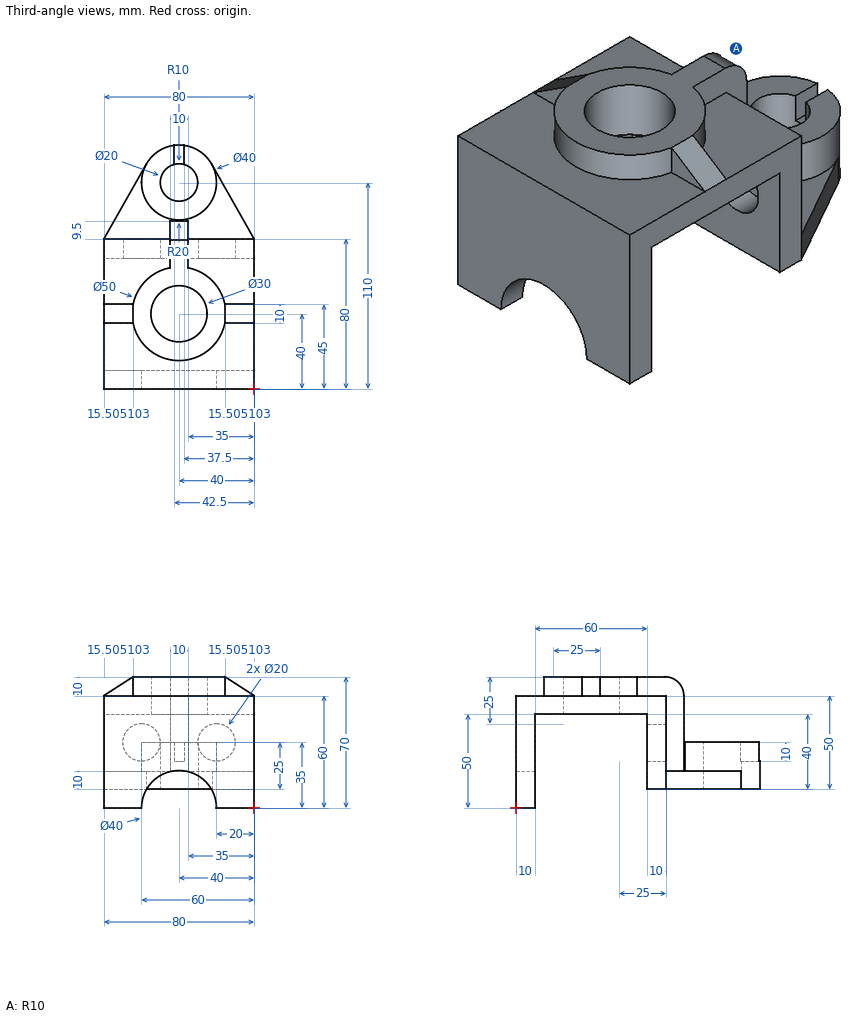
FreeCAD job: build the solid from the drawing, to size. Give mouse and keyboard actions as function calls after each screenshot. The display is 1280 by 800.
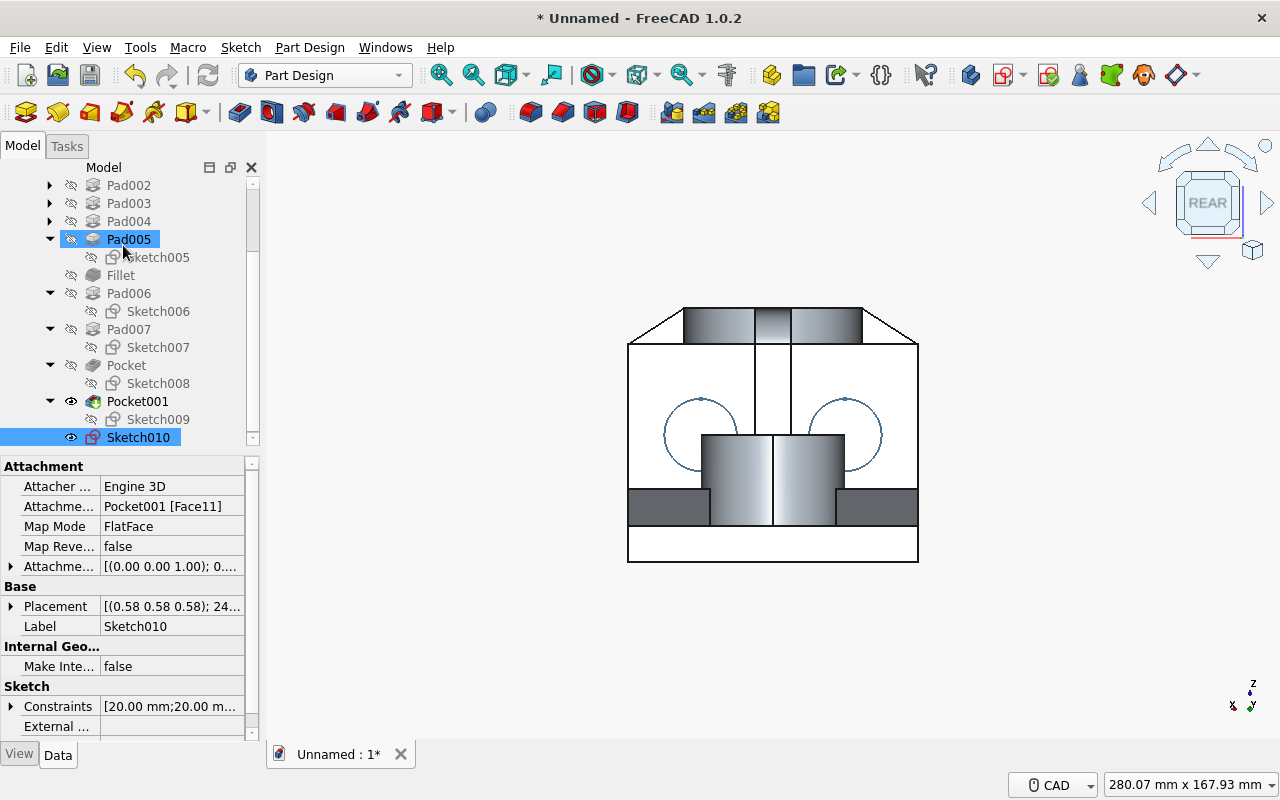
click(240, 112)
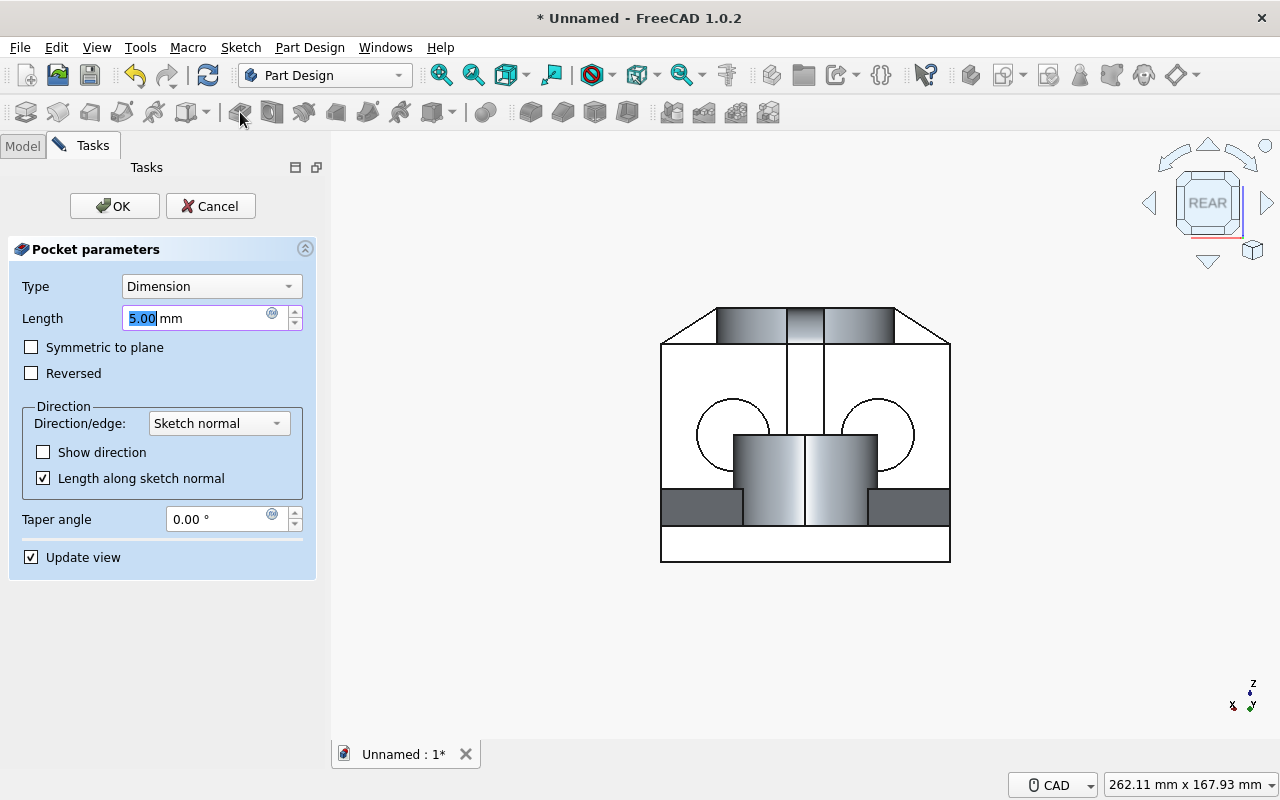
text(25)
key(Tab)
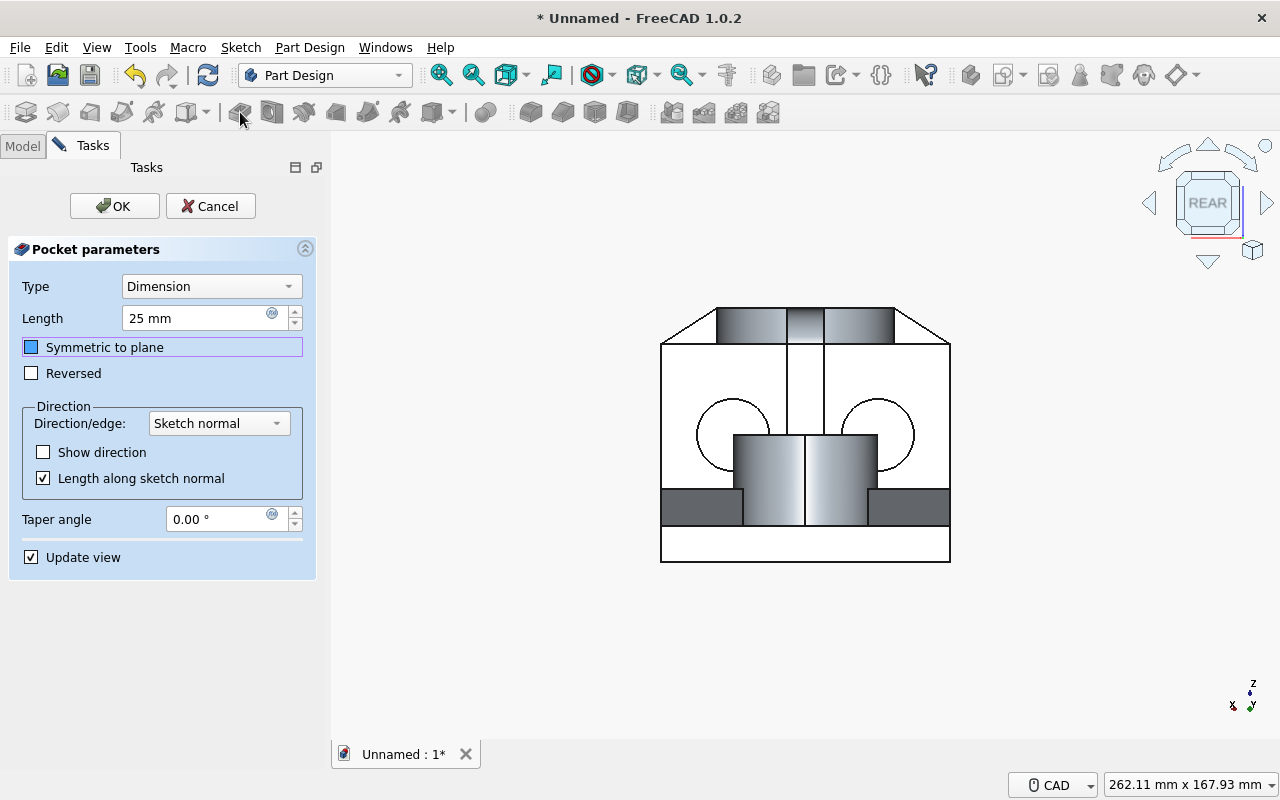
click(115, 206)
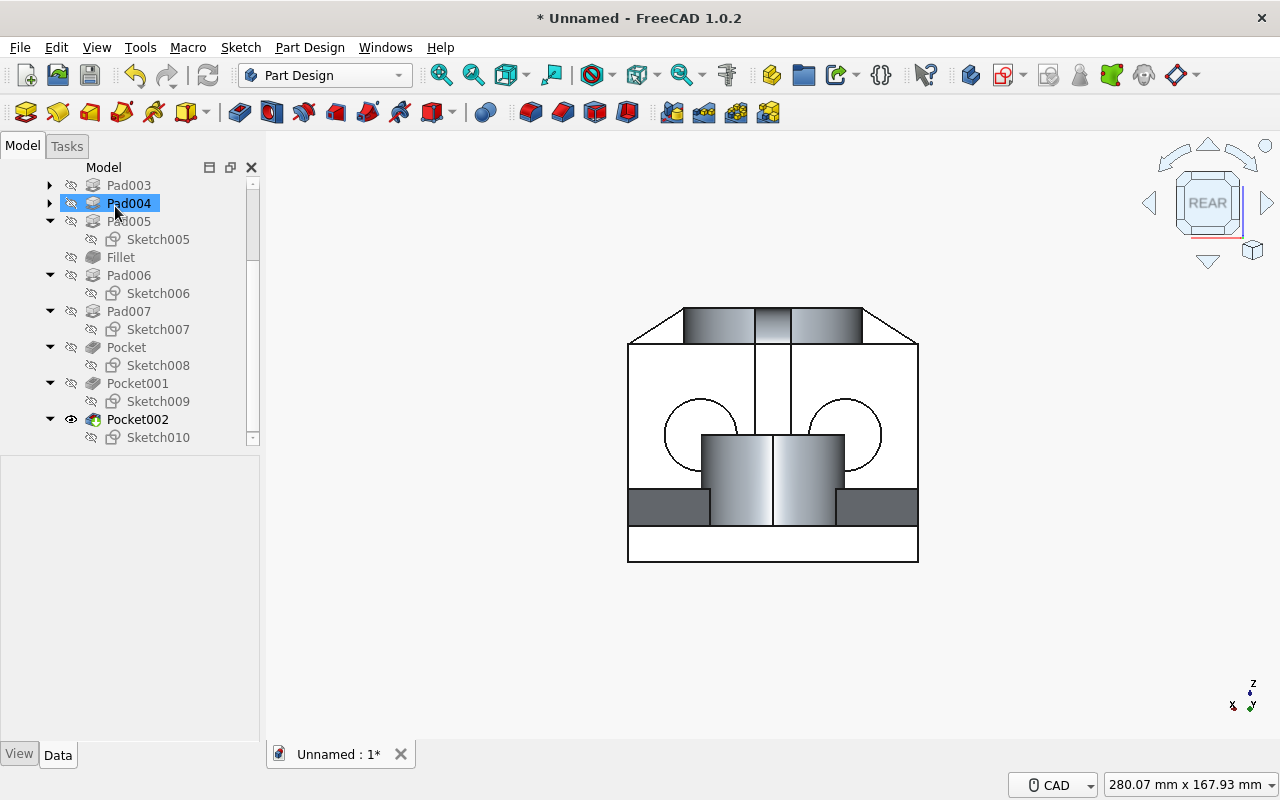
click(442, 76)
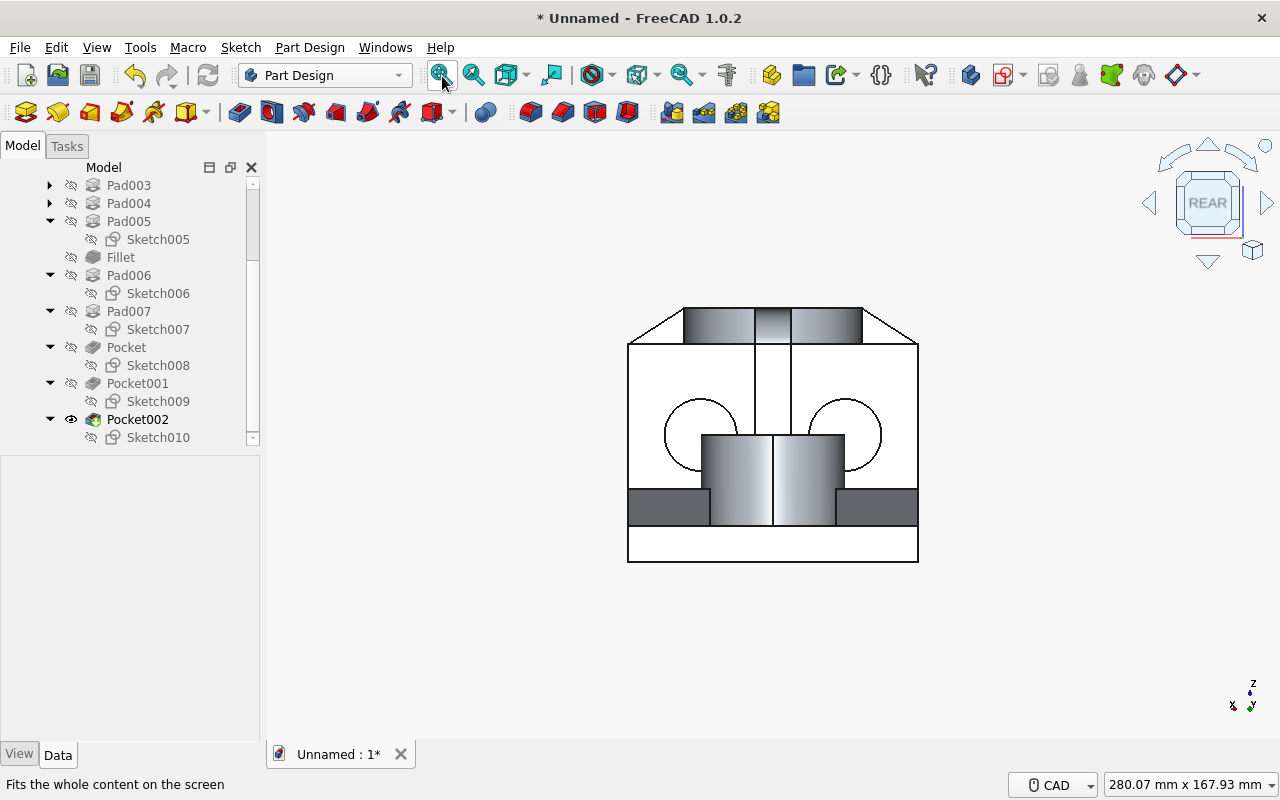
key(0)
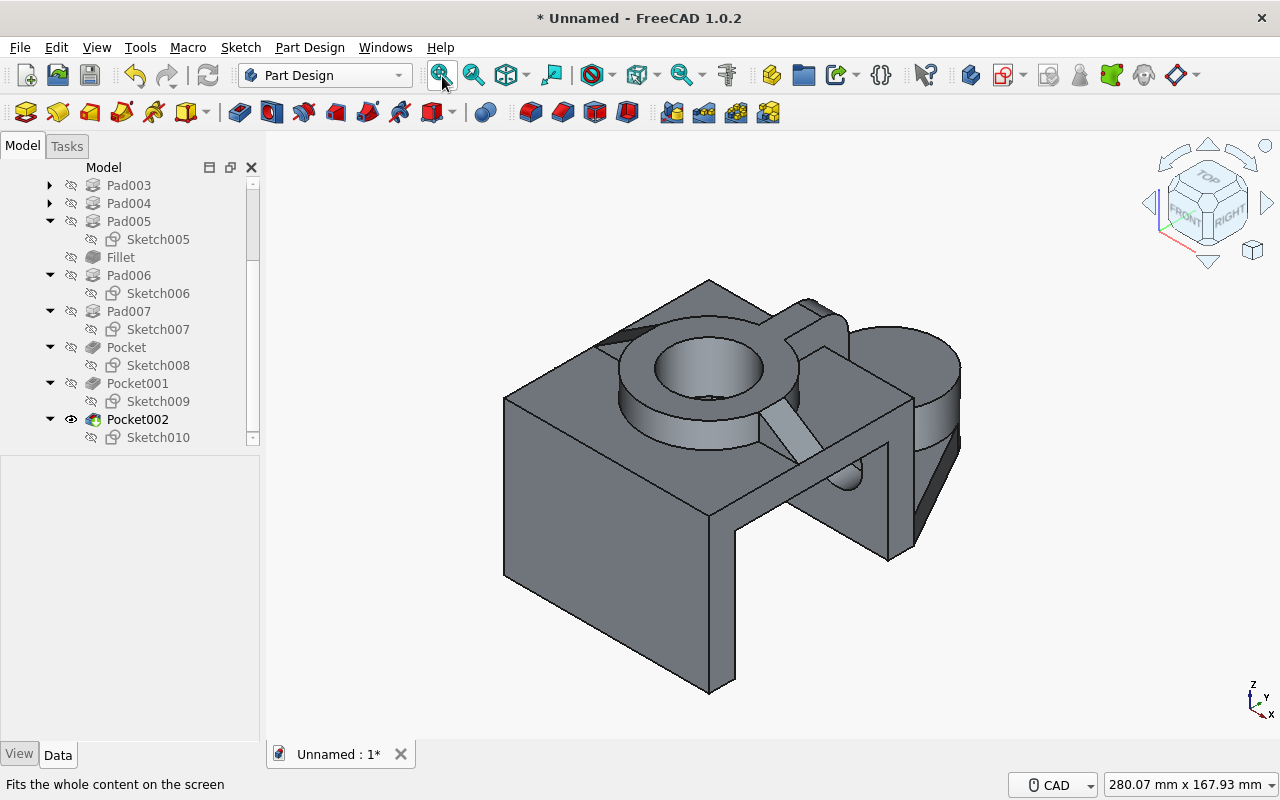
click(888, 367)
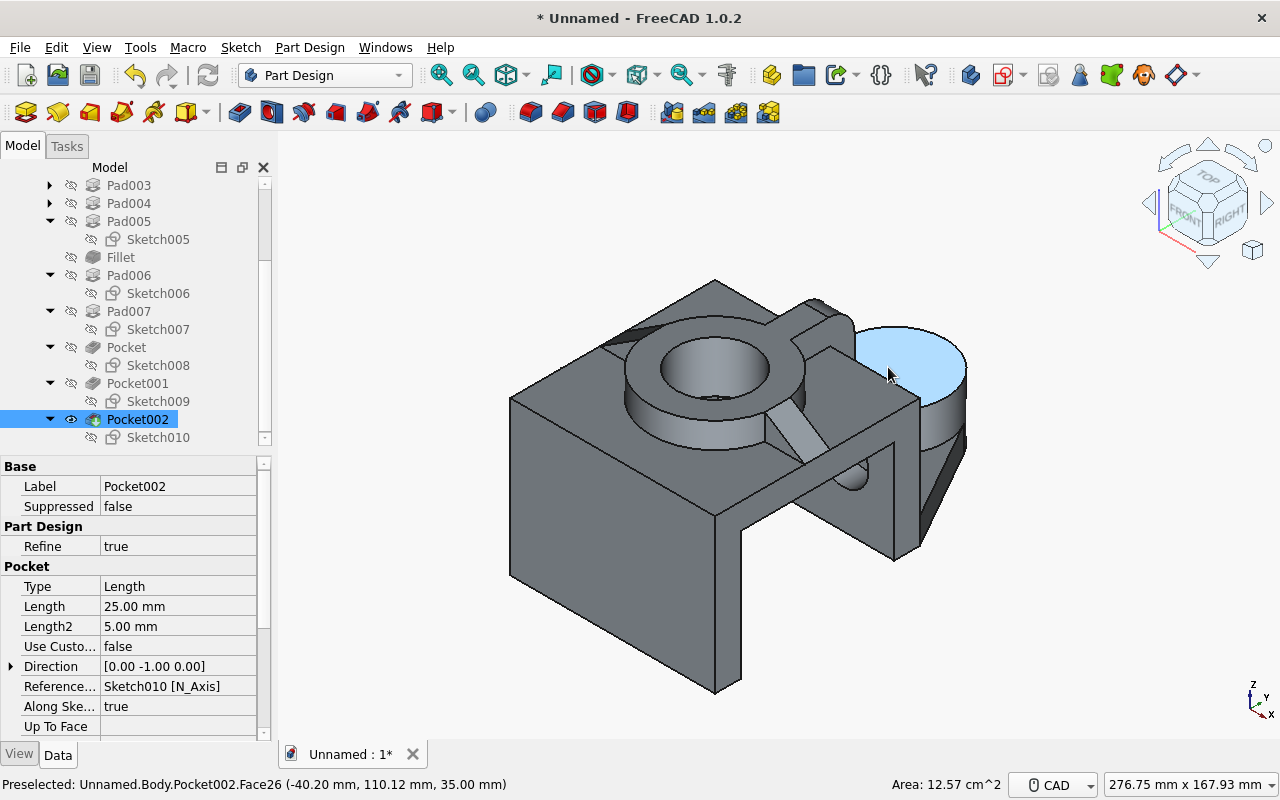
click(1004, 76)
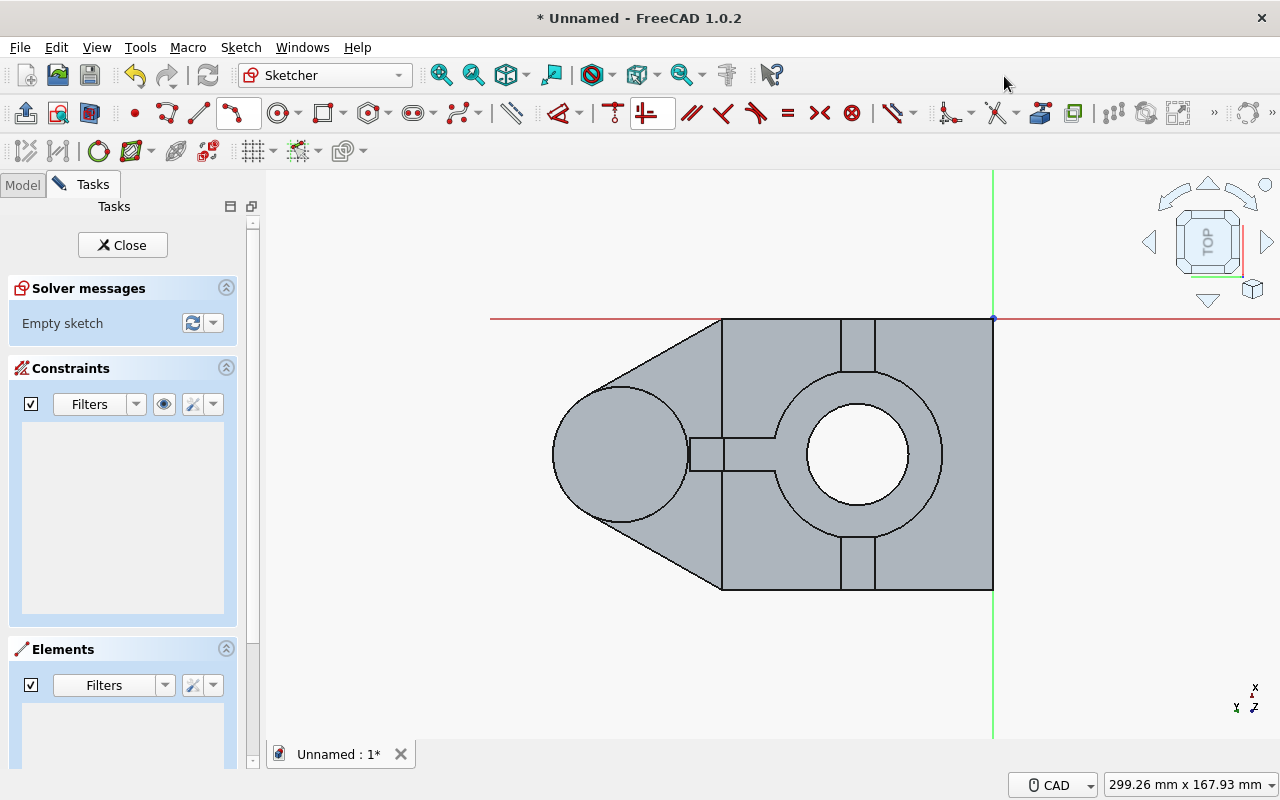
scroll(599, 455, up, 8)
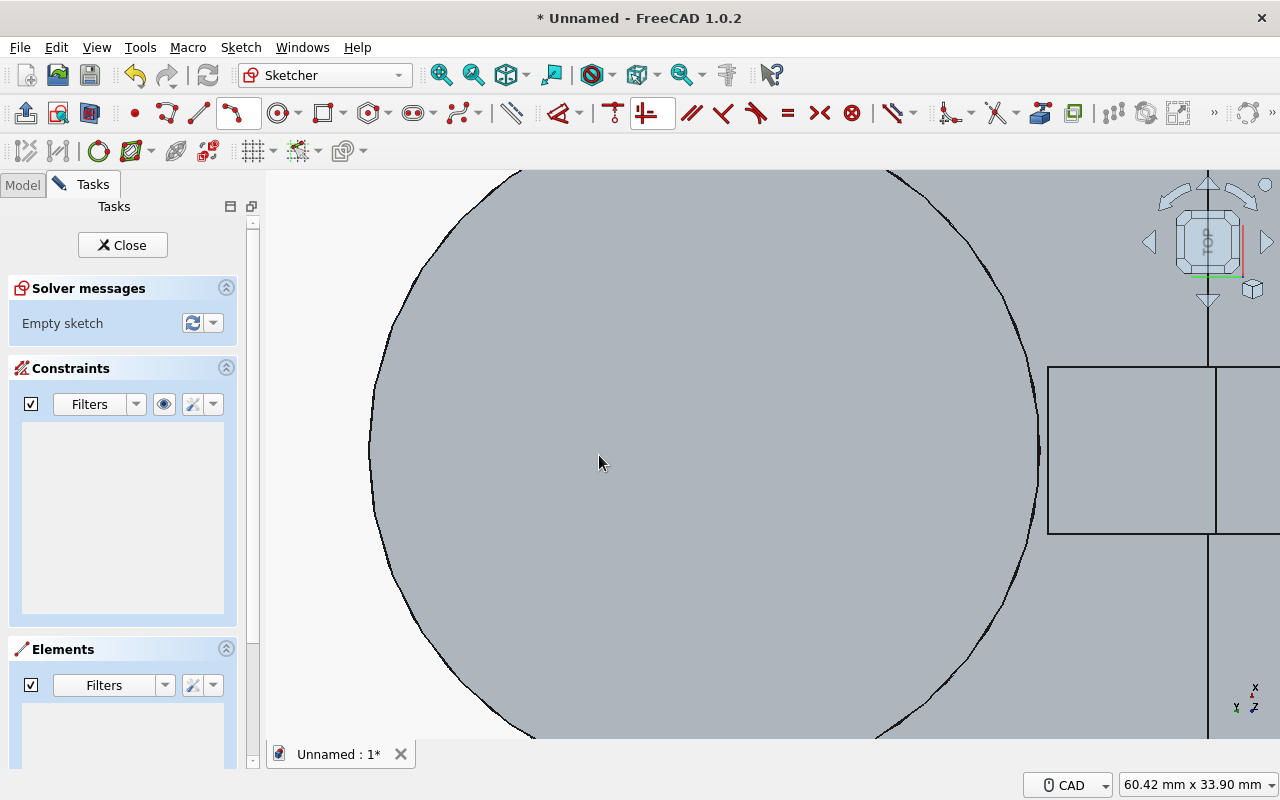
click(278, 114)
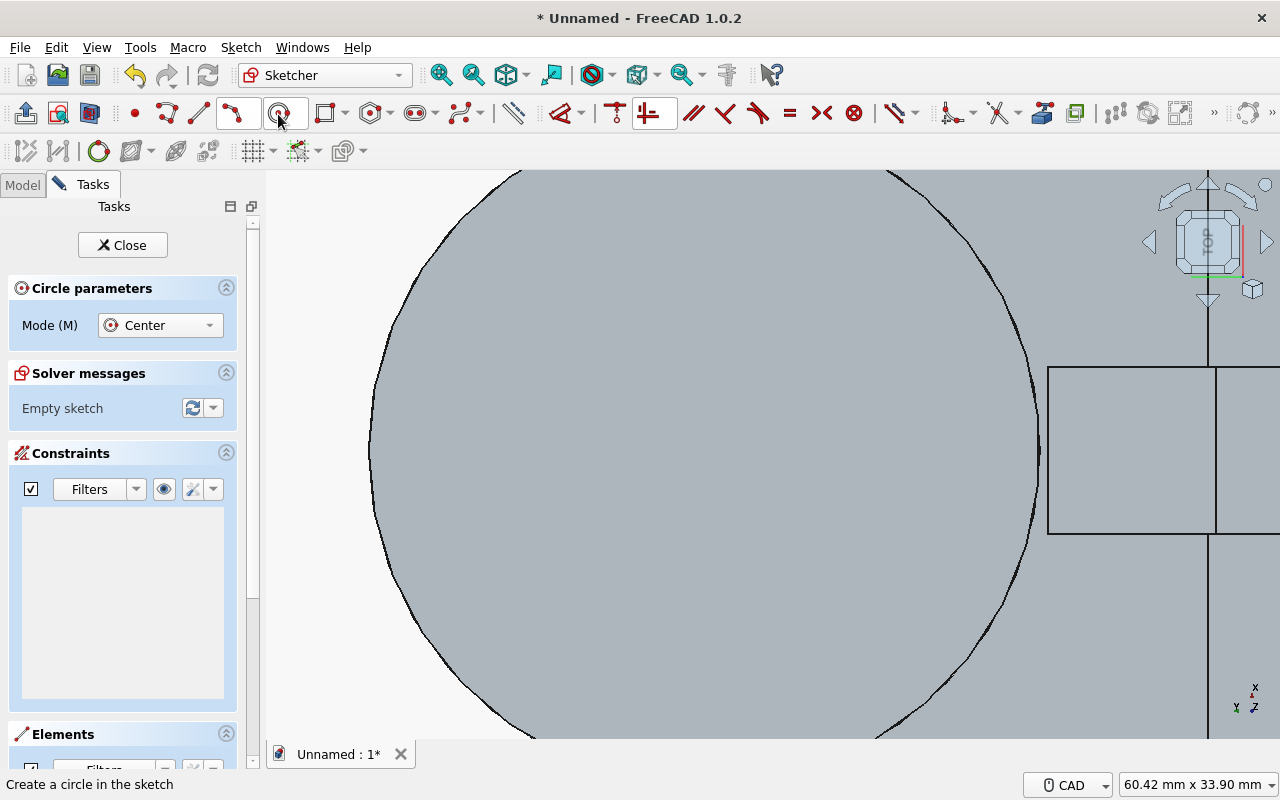
click(704, 451)
move(823, 332)